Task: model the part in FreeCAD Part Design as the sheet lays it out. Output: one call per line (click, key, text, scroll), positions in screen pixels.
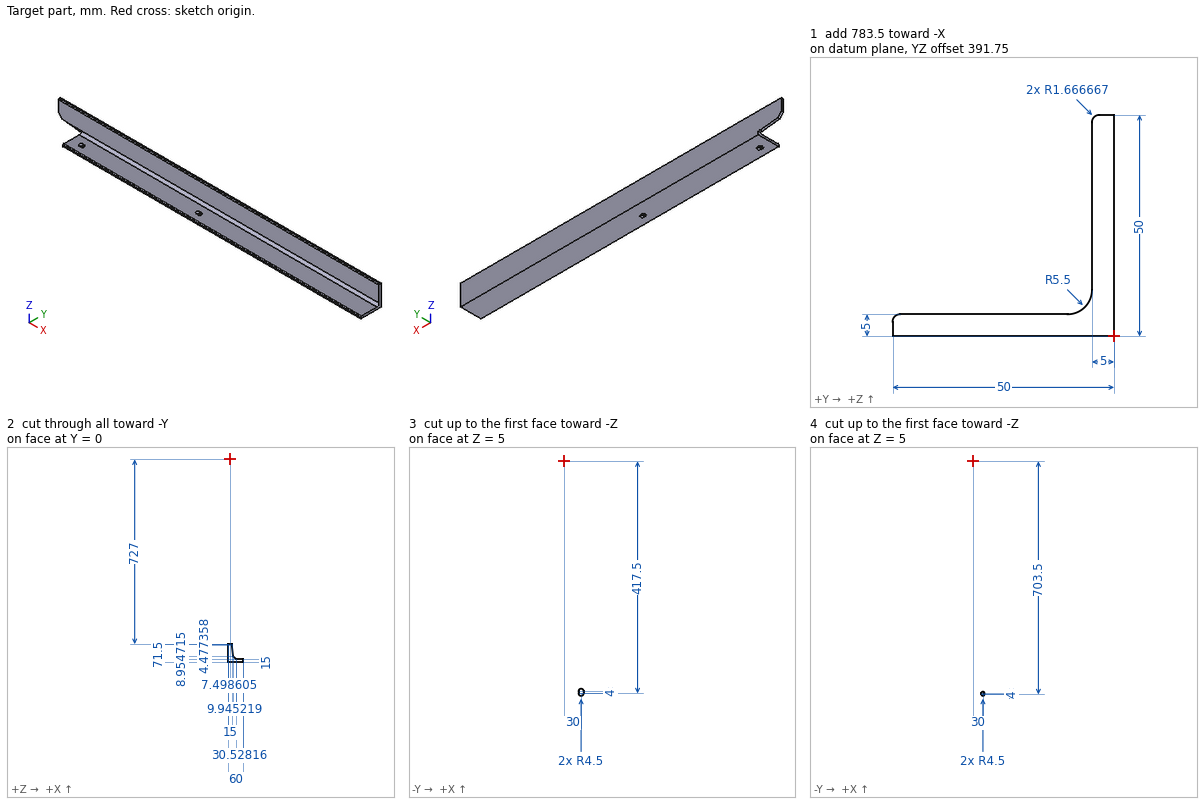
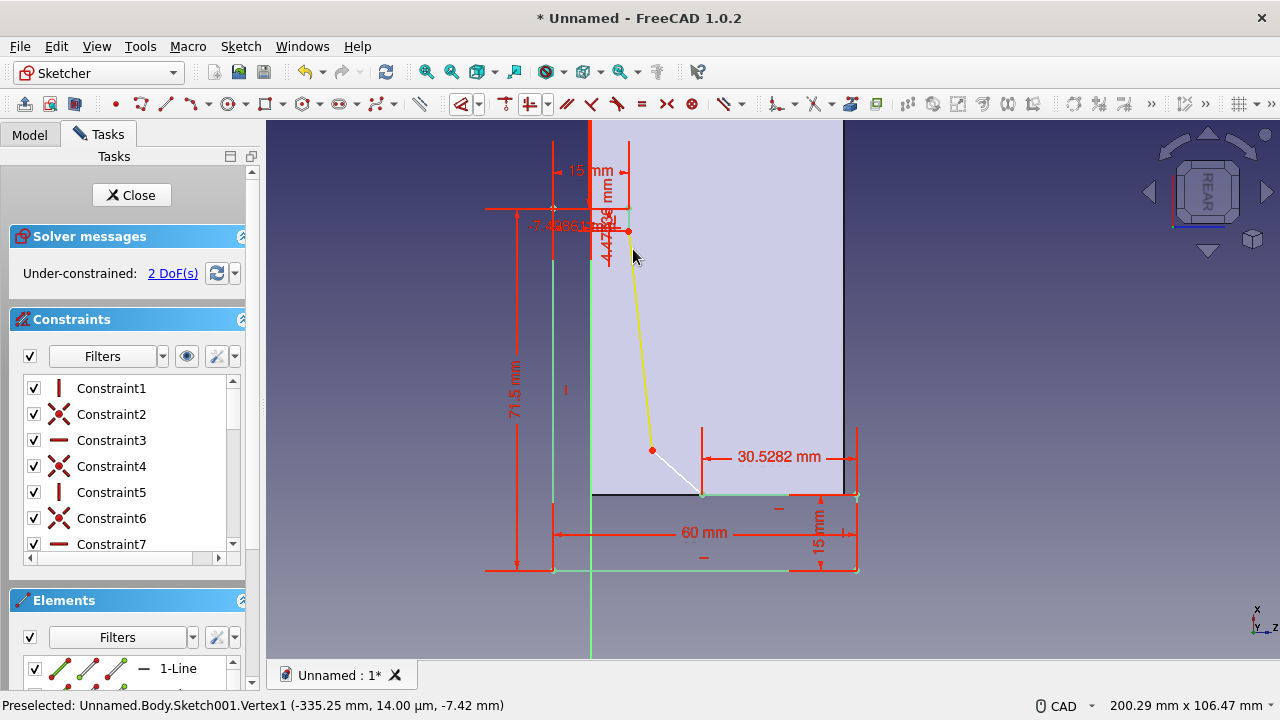
click(687, 481)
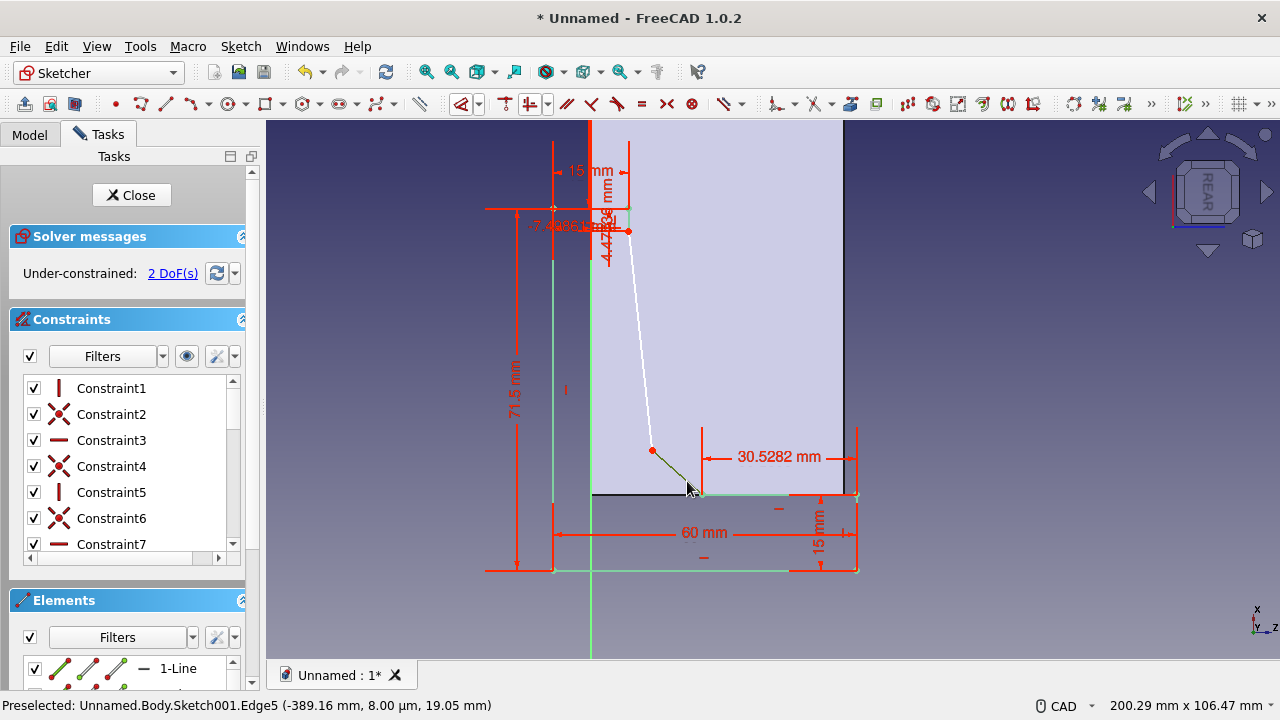
click(478, 104)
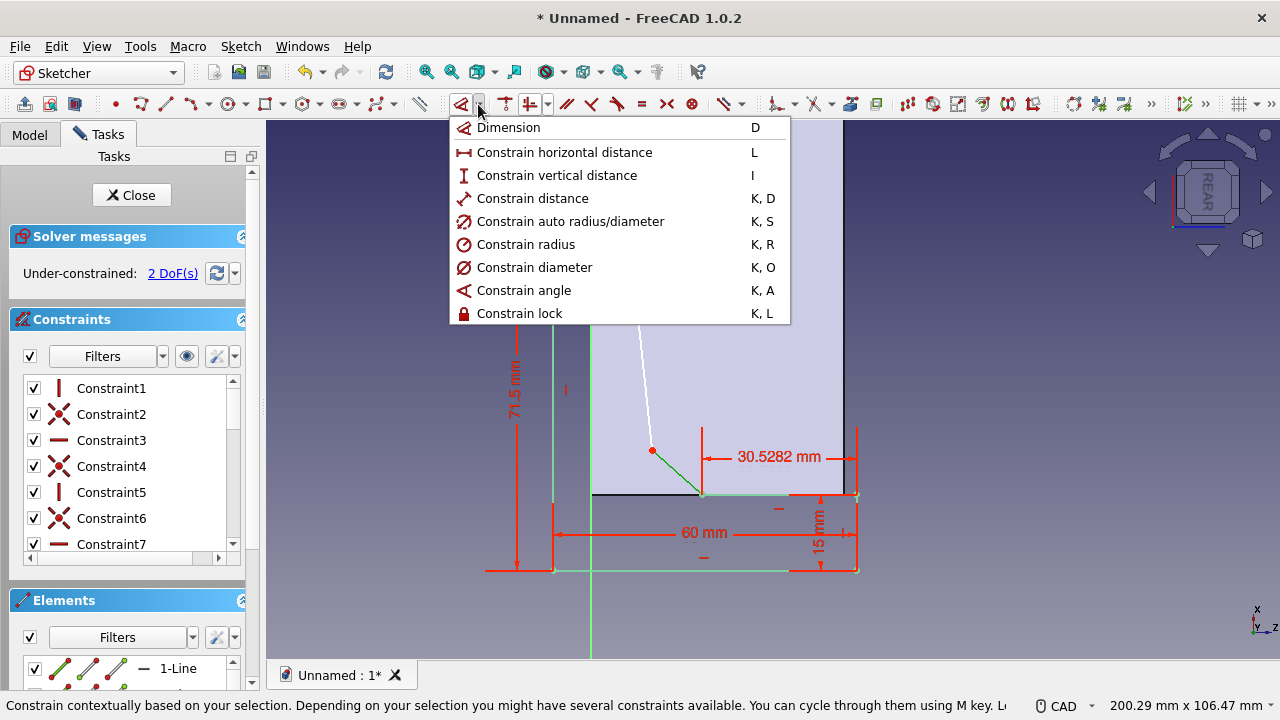
click(620, 152)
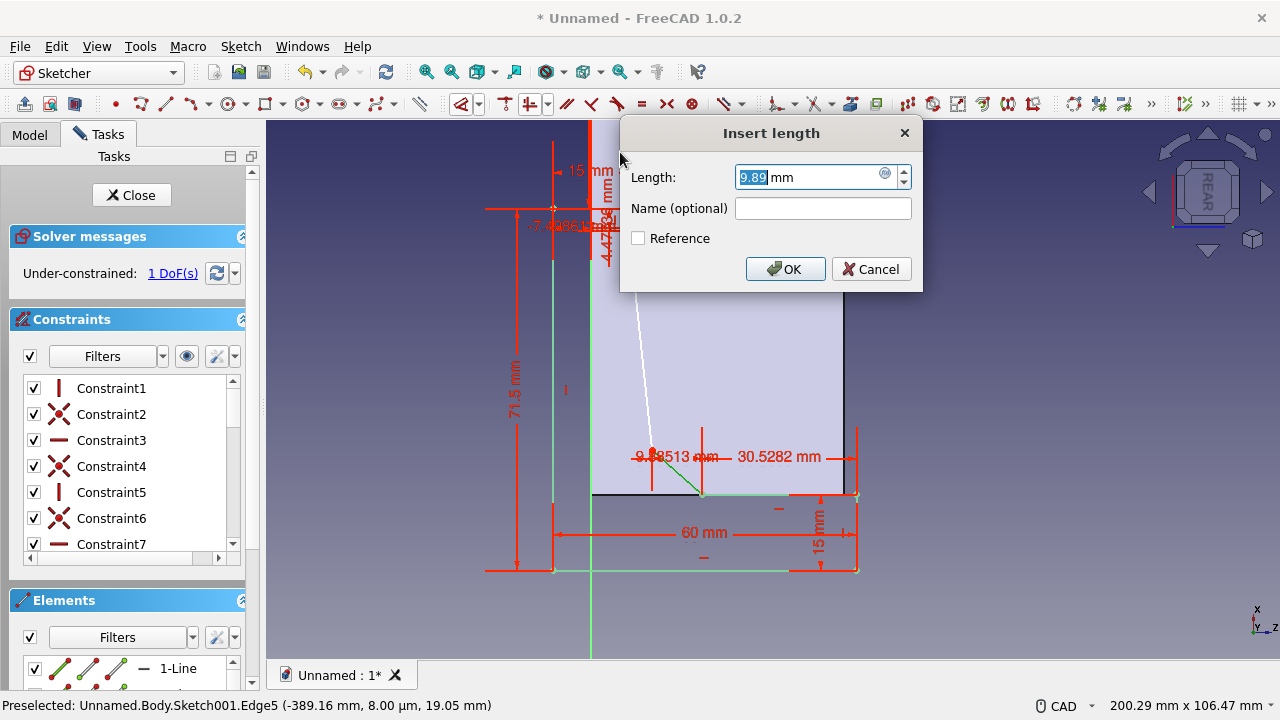
text(9.945219)
key(Return)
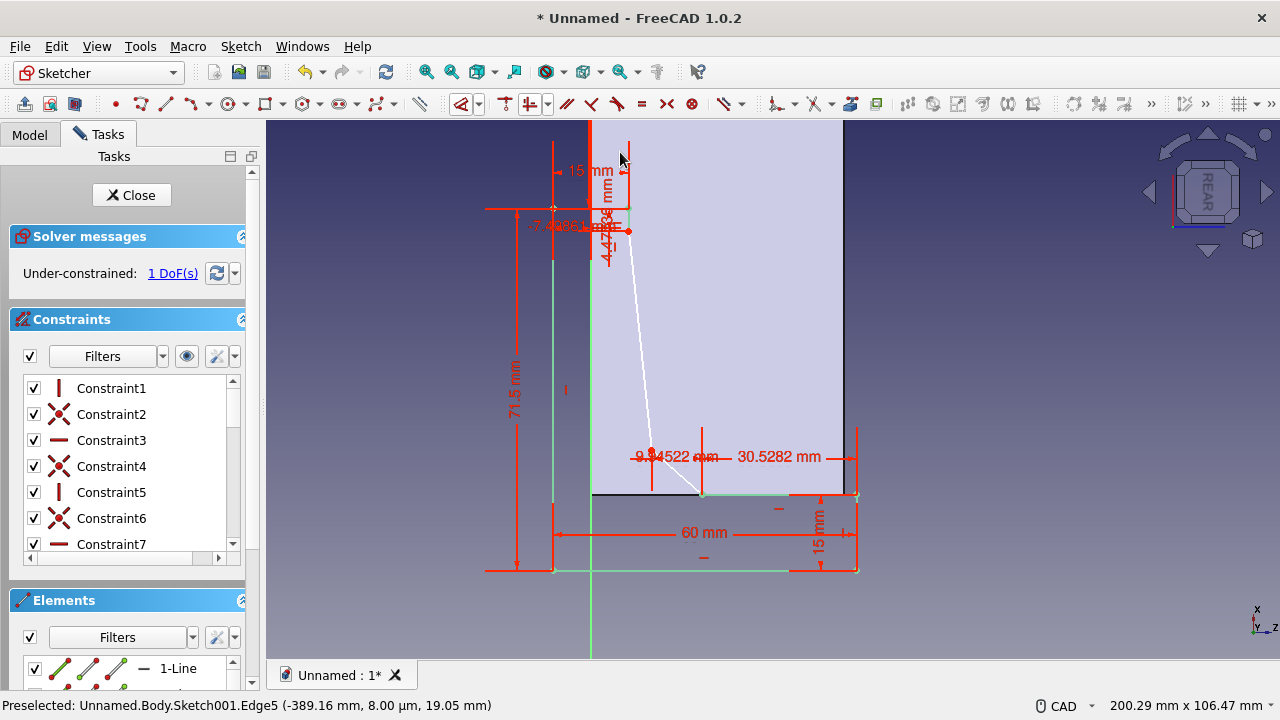
click(687, 481)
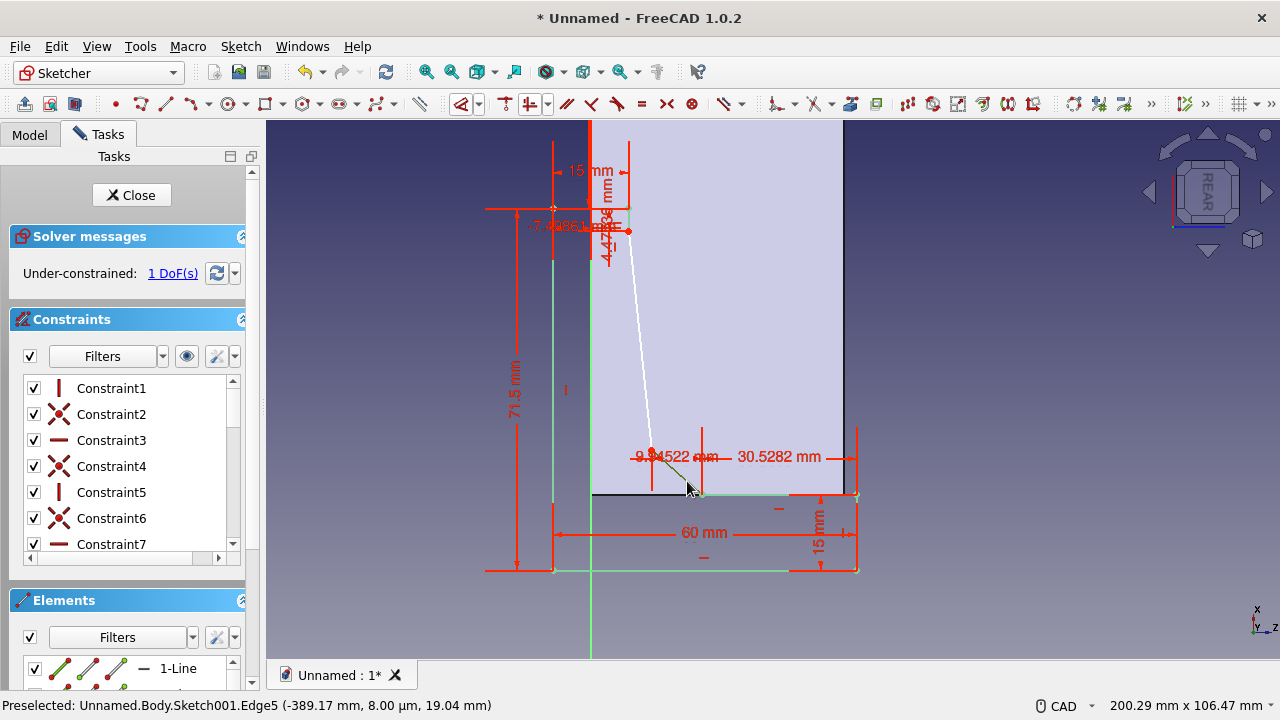
click(478, 104)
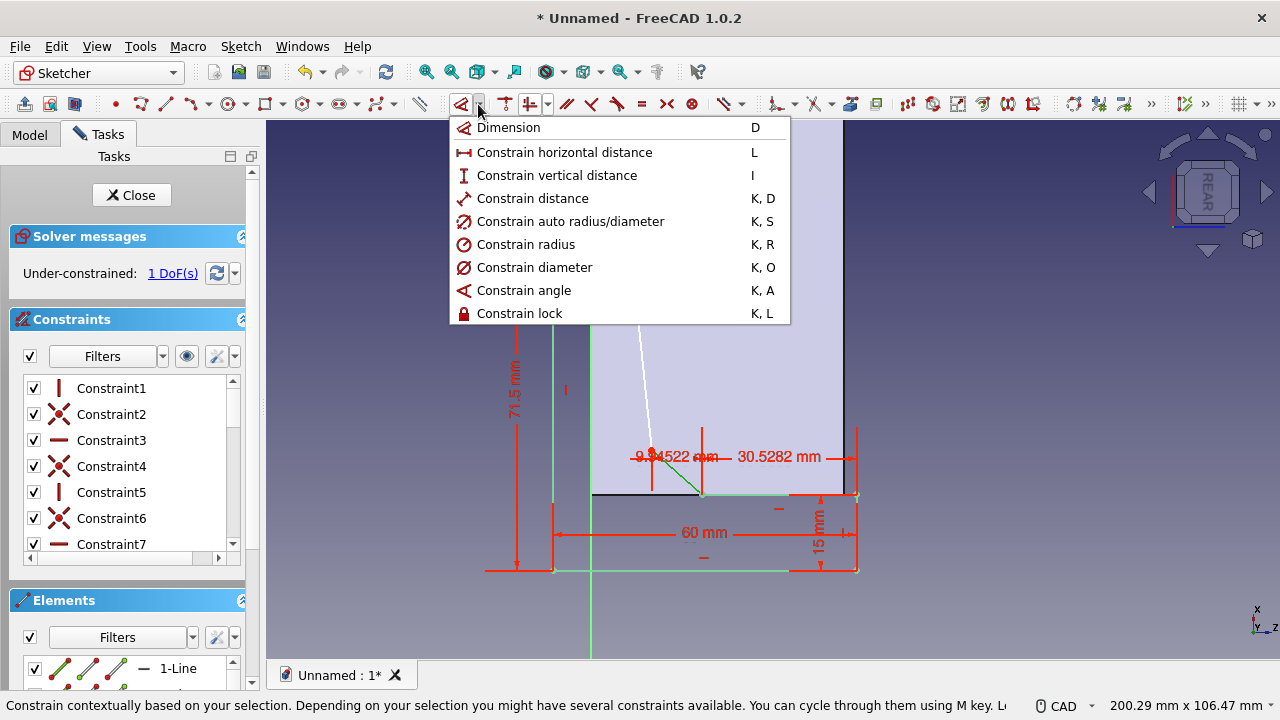
click(620, 176)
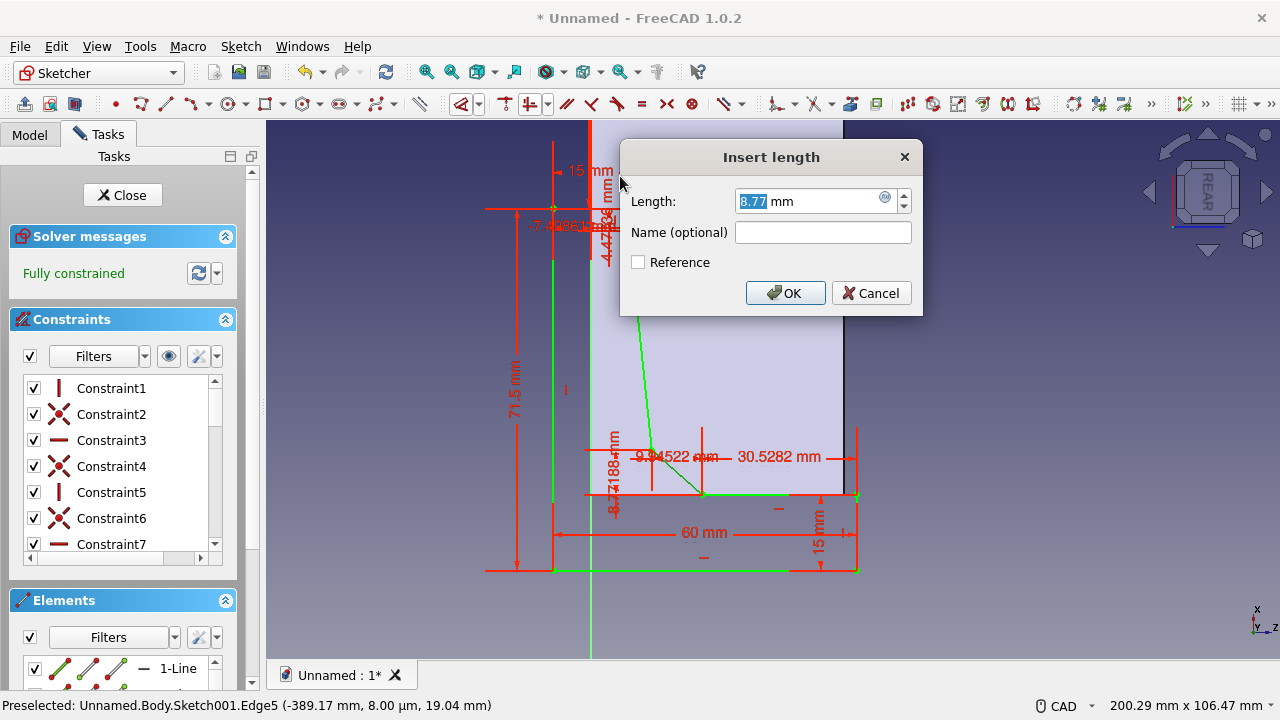
text(8.954715)
key(Return)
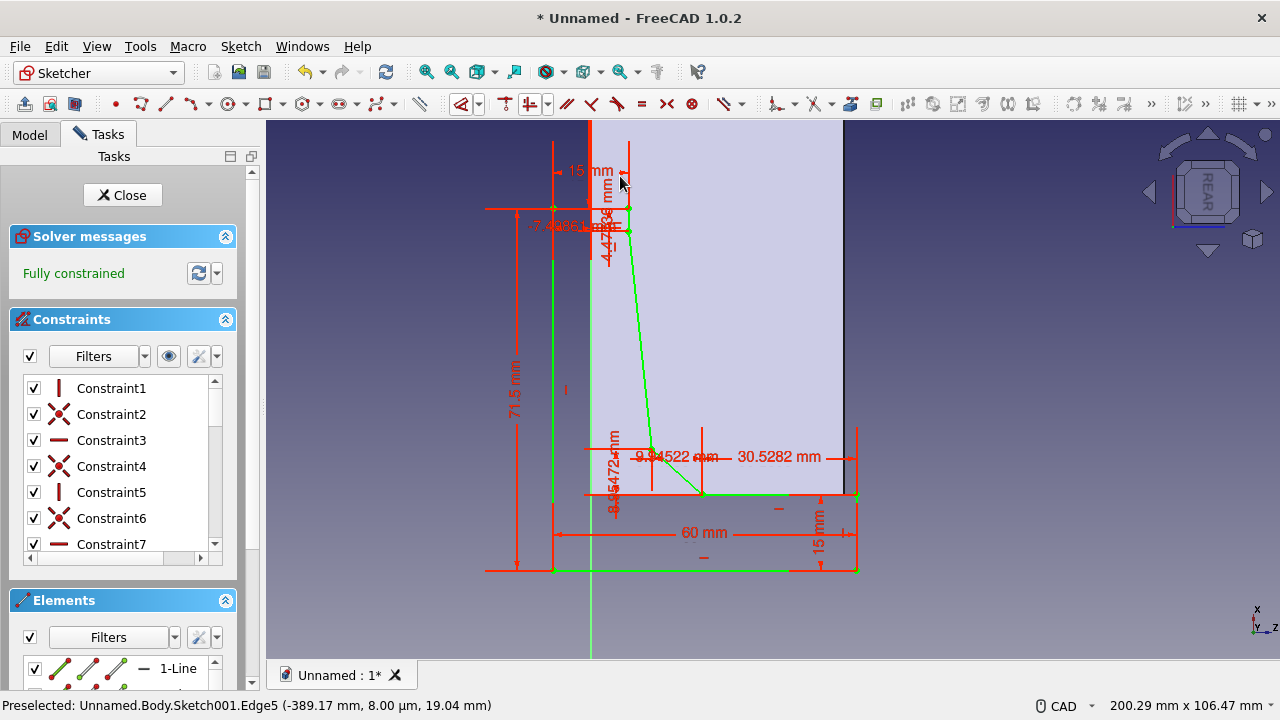
click(123, 195)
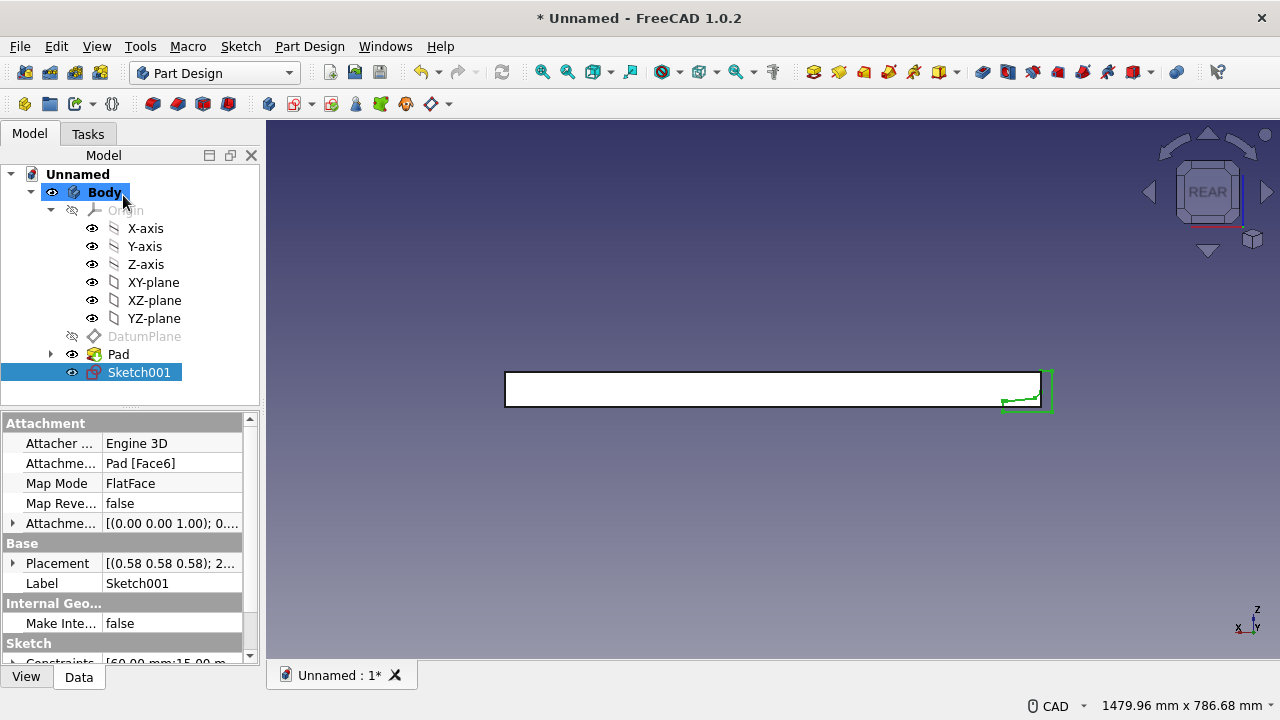
click(983, 72)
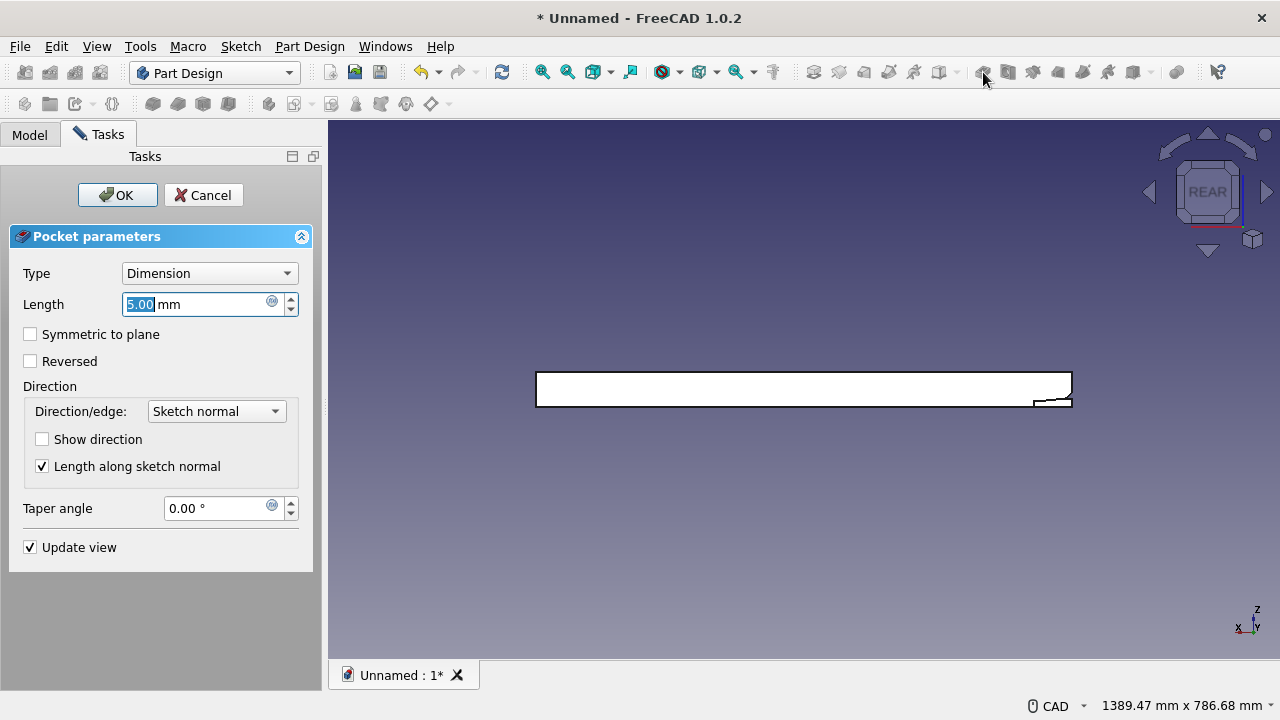
click(210, 274)